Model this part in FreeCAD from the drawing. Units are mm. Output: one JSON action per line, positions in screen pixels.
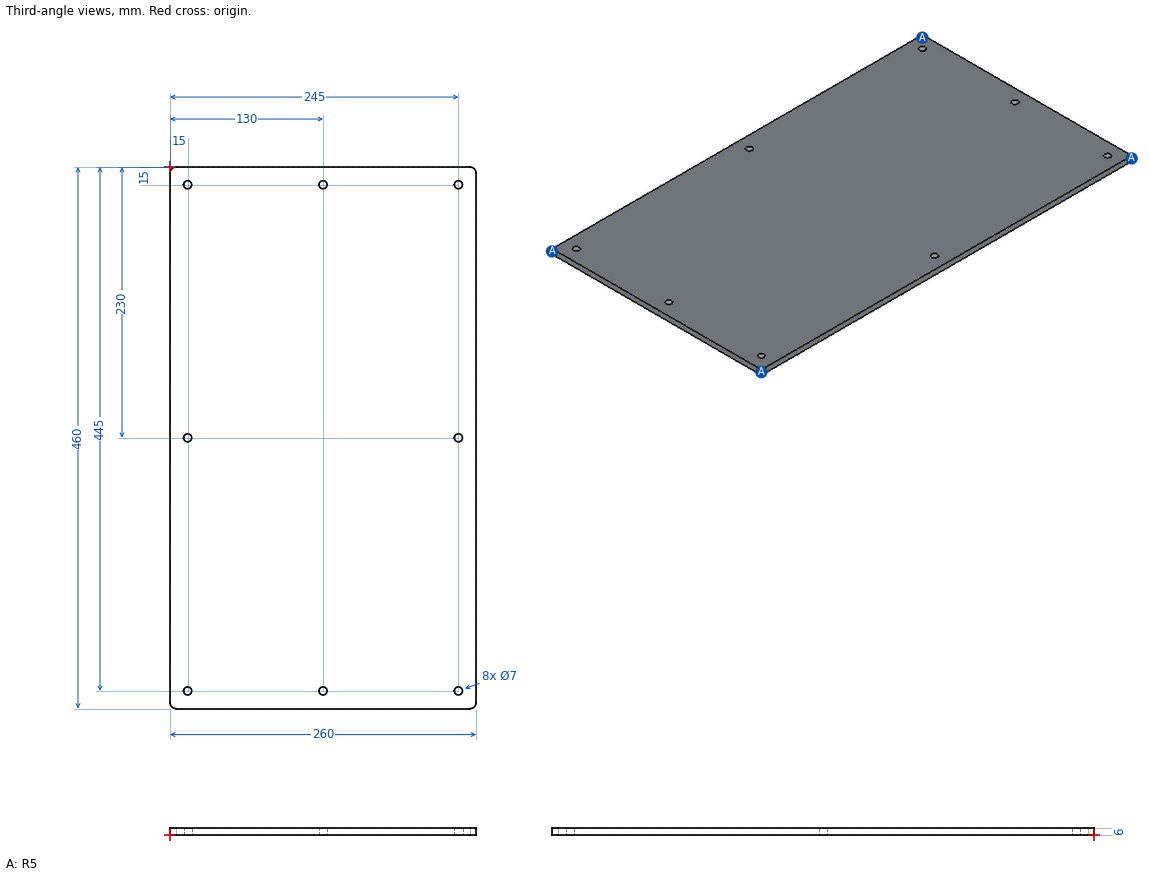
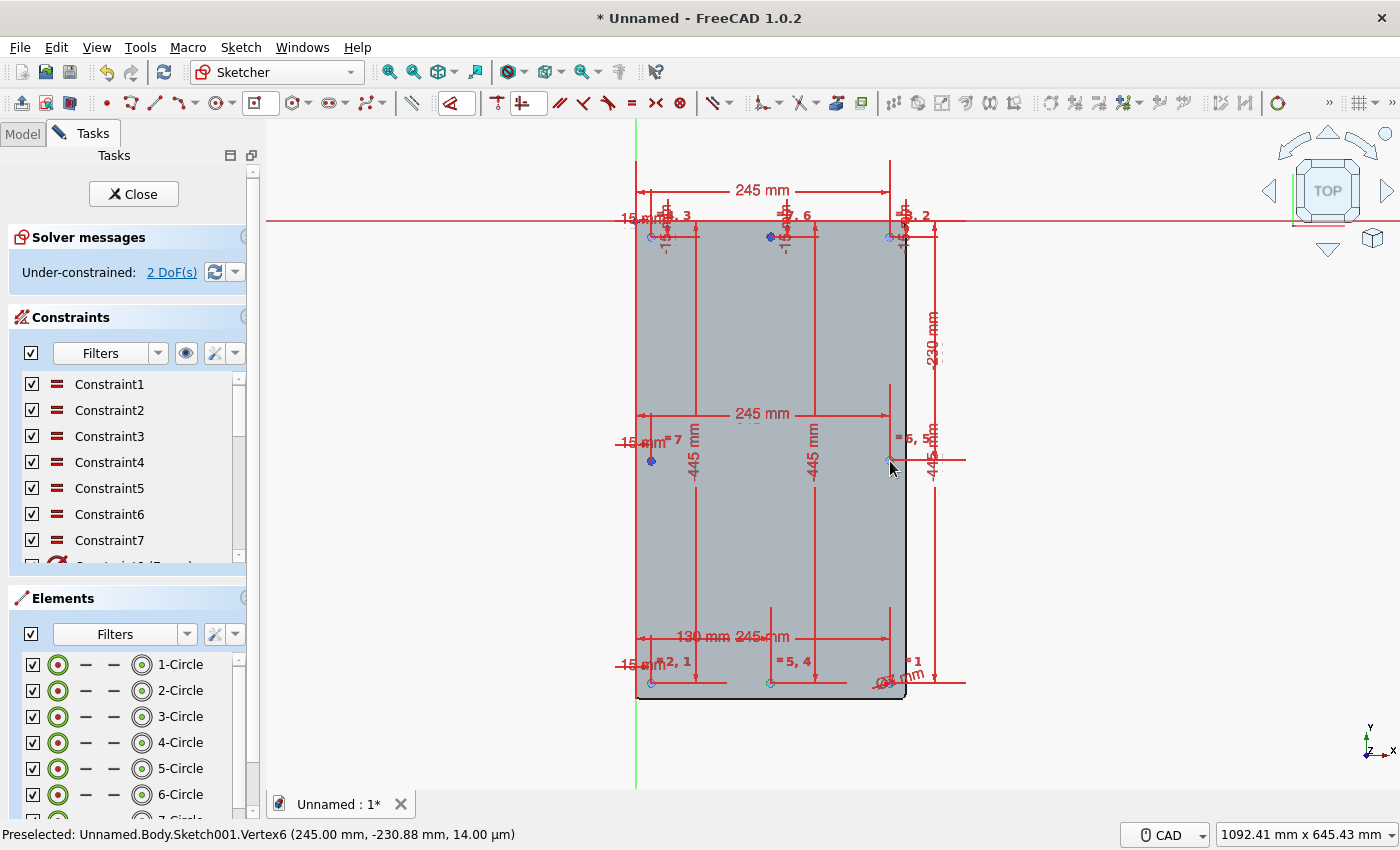
{"action": "left_click", "coordinate": [771, 237]}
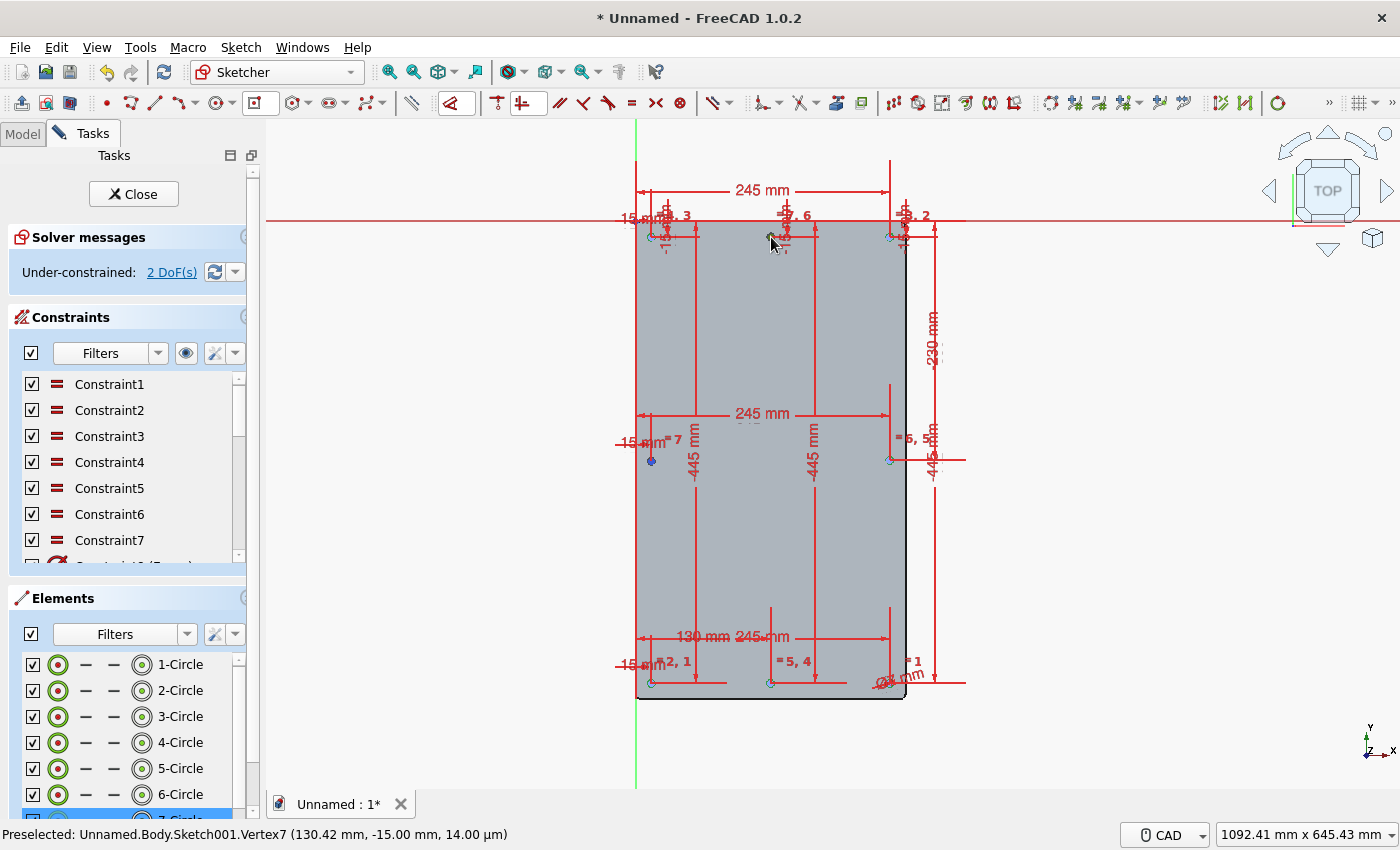
{"action": "key", "text": "l"}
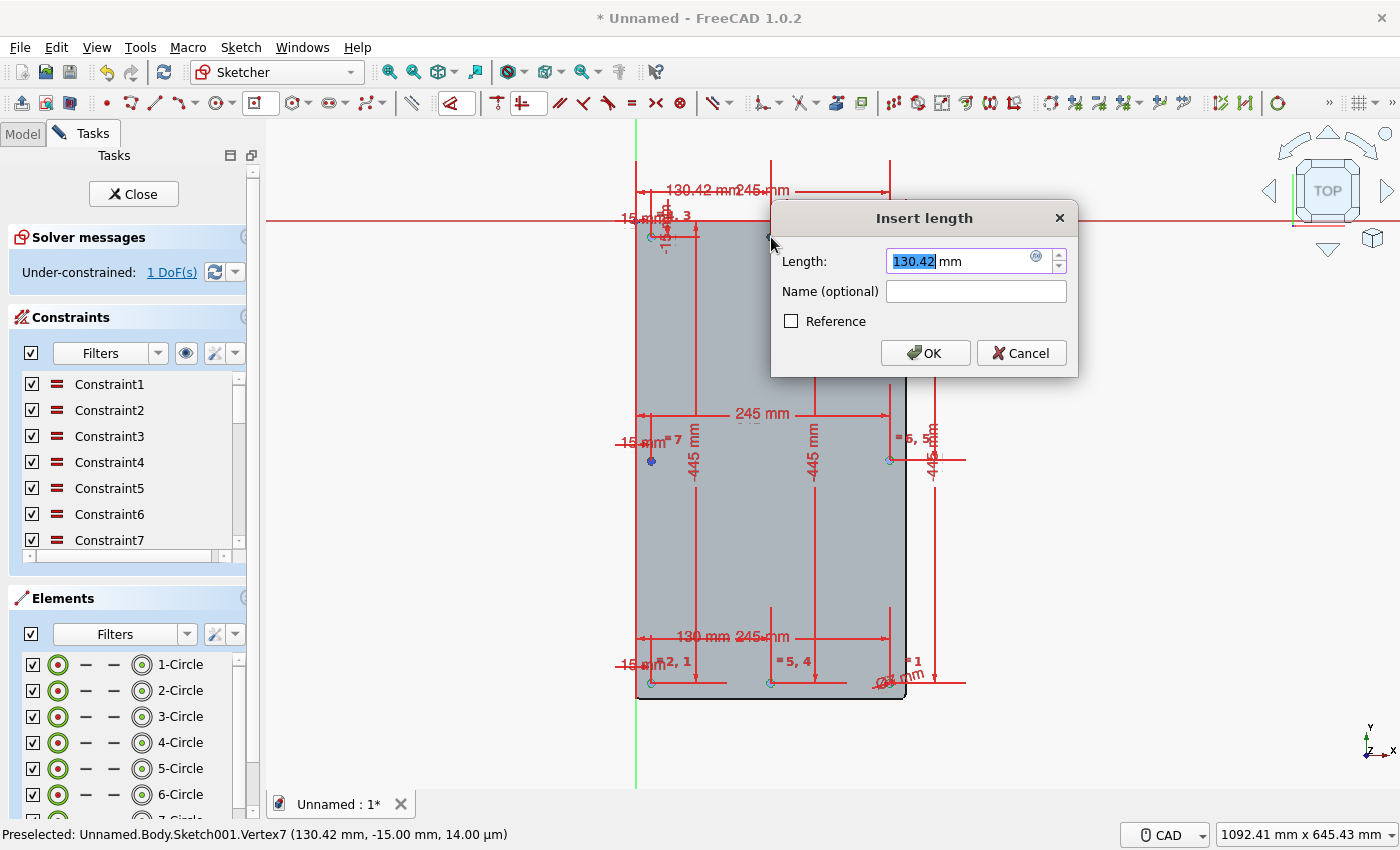
{"action": "type", "text": "130"}
{"action": "key", "text": "Return"}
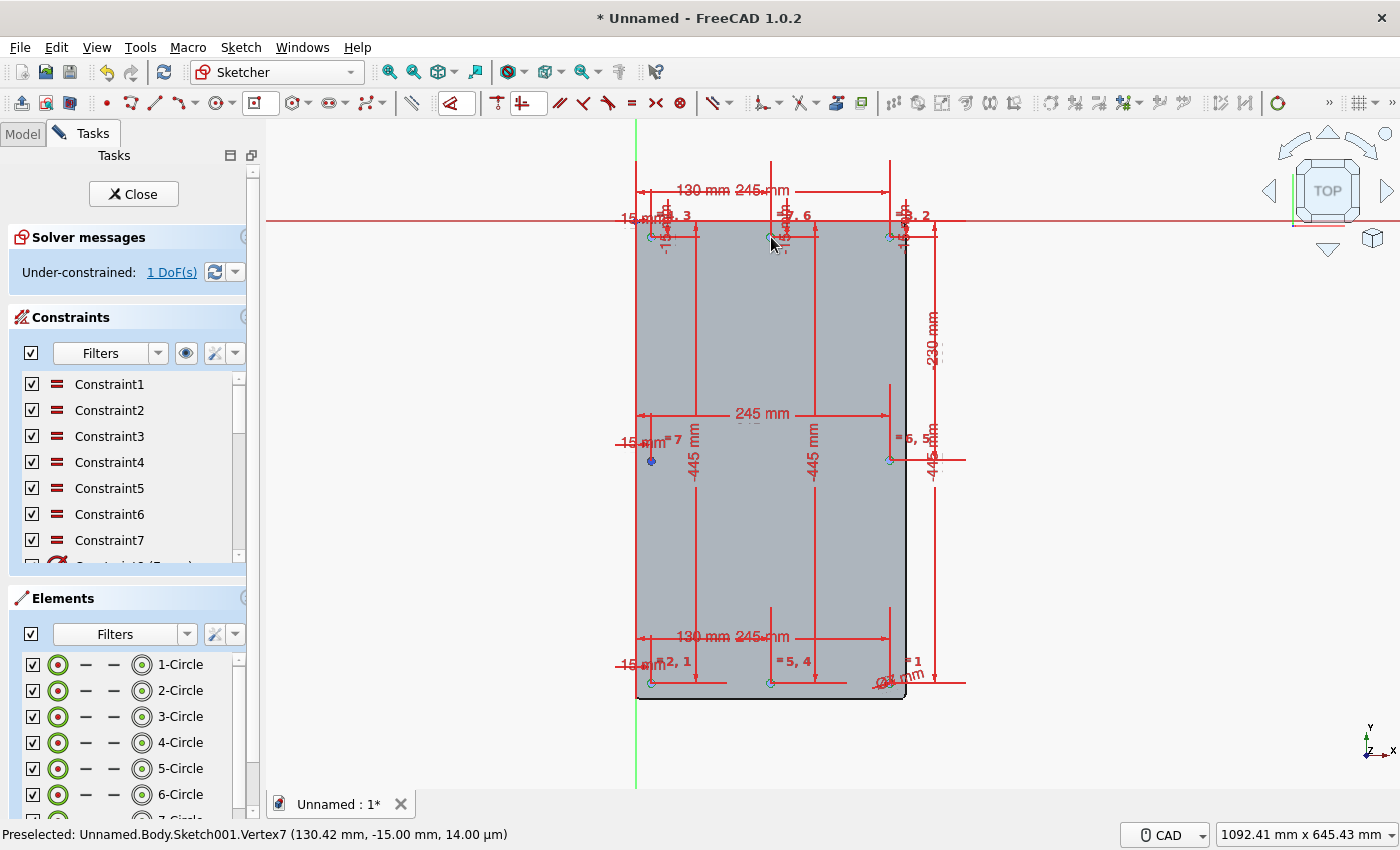
{"action": "left_click", "coordinate": [651, 461]}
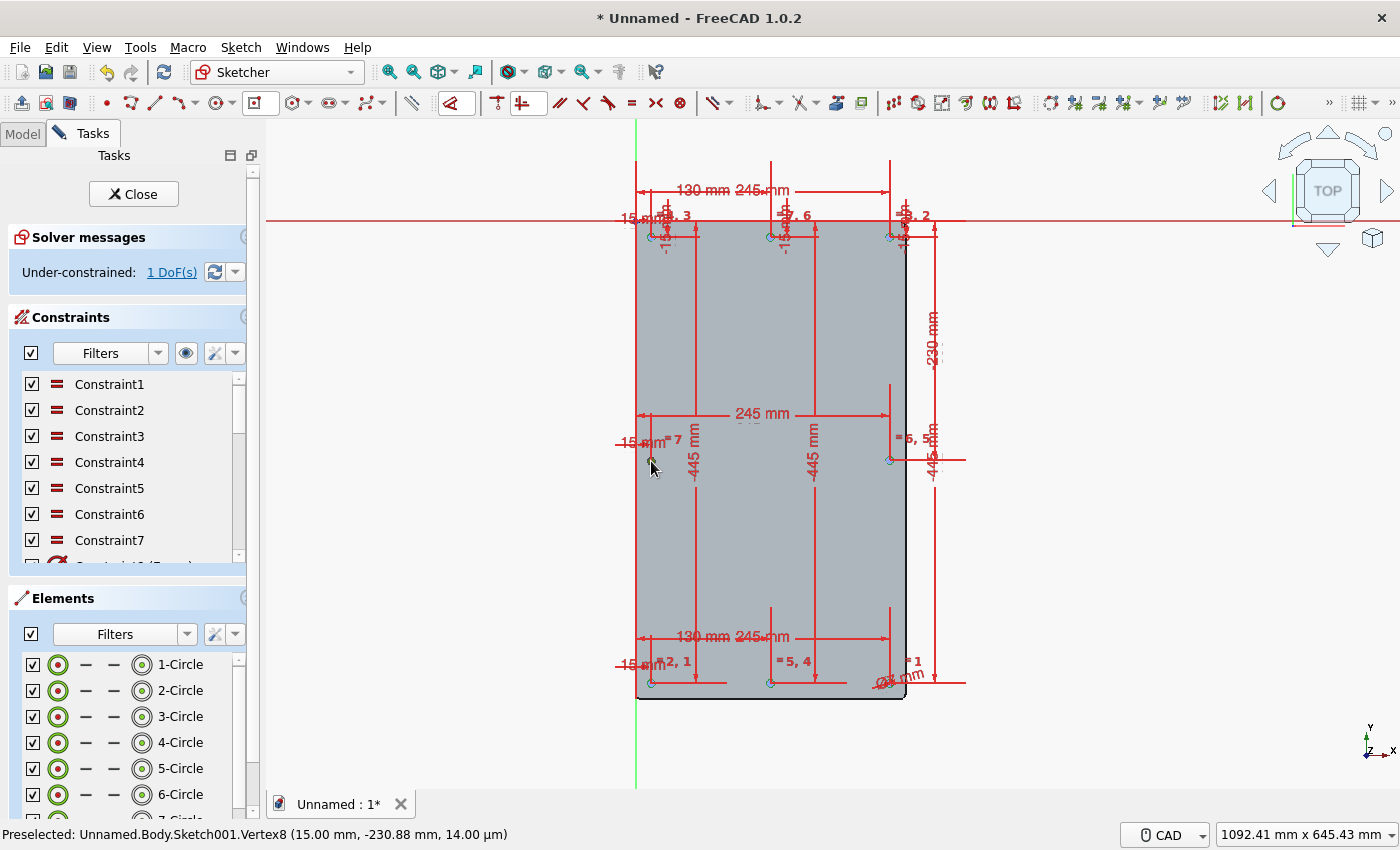
{"action": "left_click", "coordinate": [470, 104]}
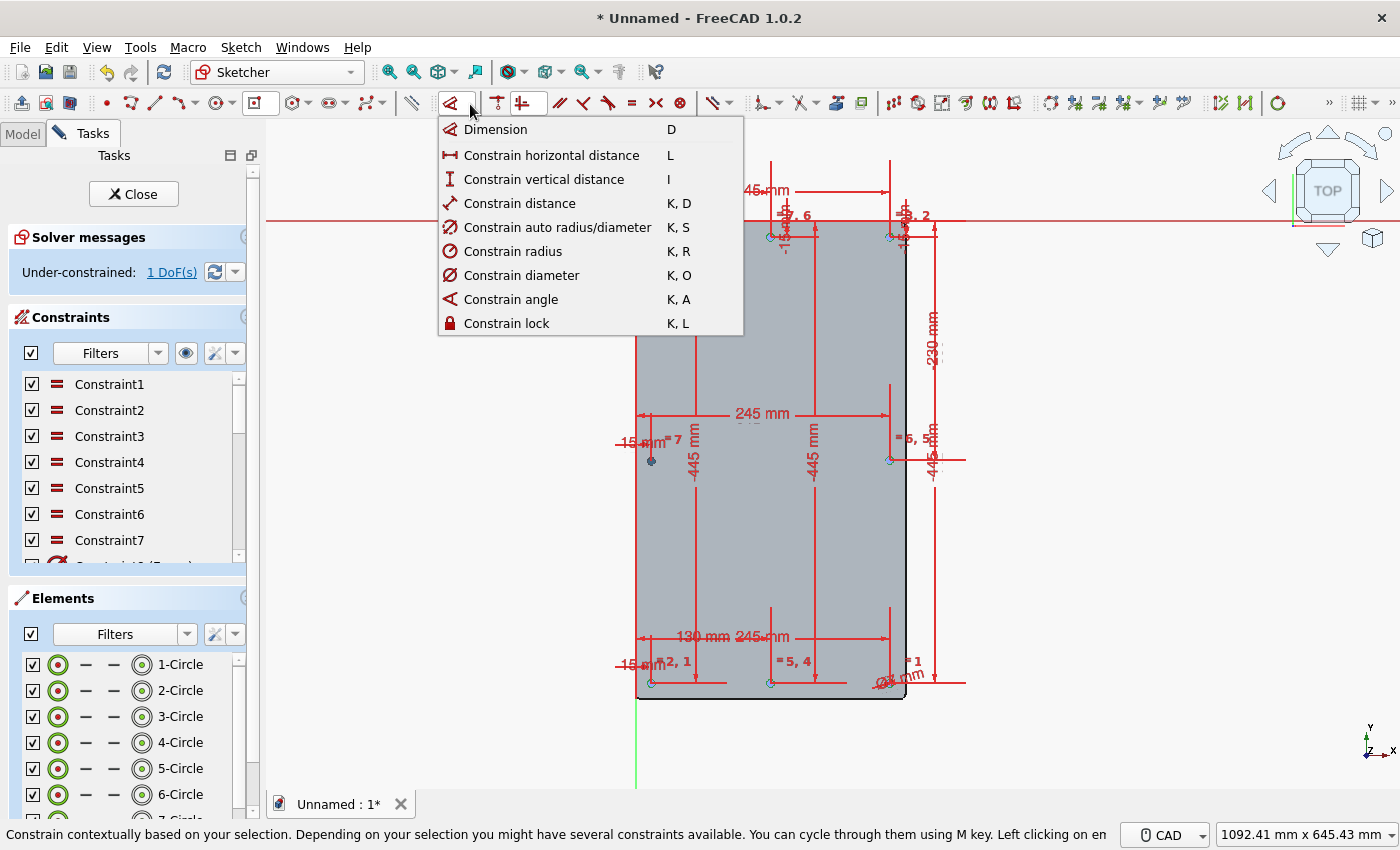
{"action": "left_click", "coordinate": [591, 179]}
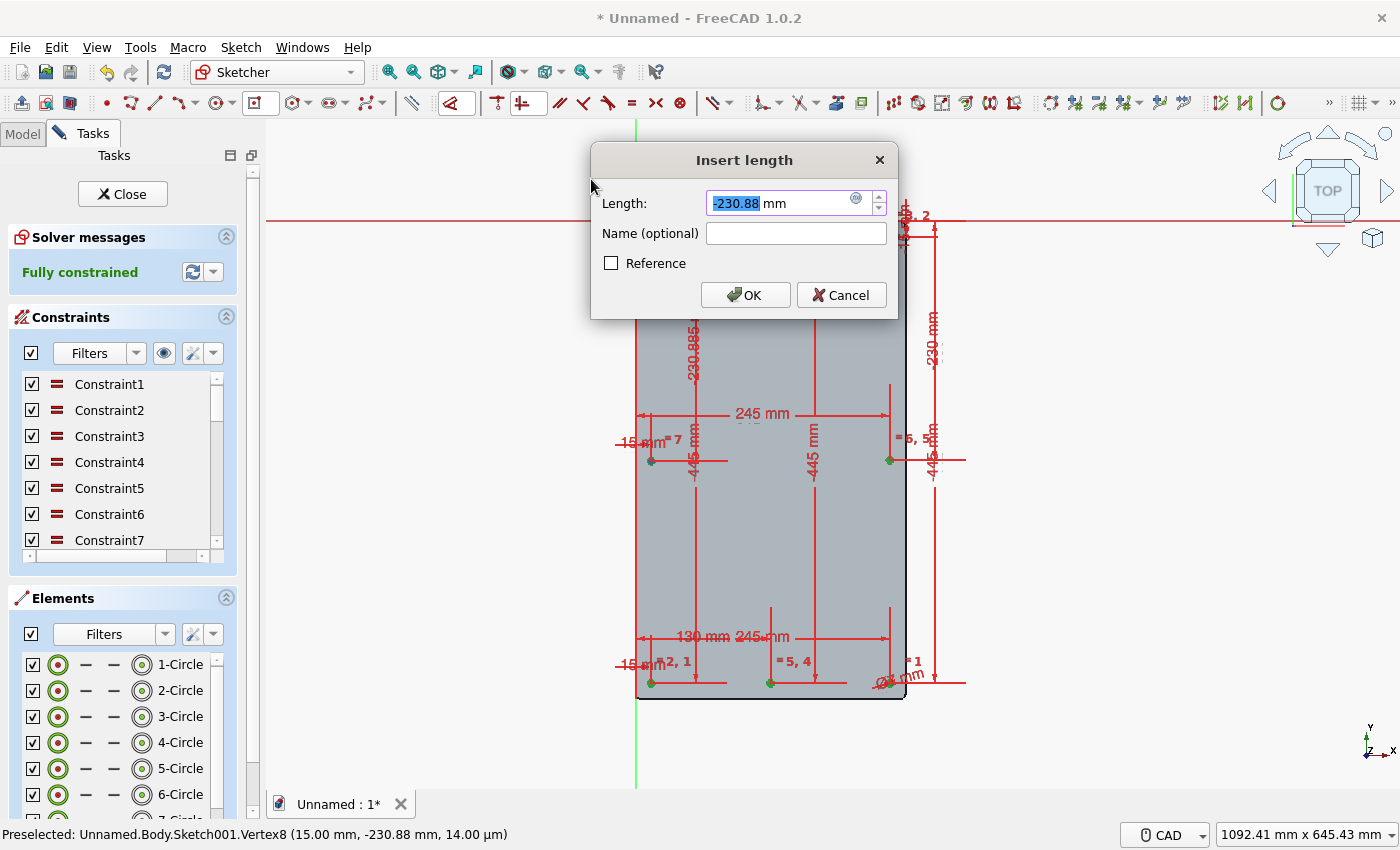
{"action": "type", "text": "-230"}
{"action": "key", "text": "Return"}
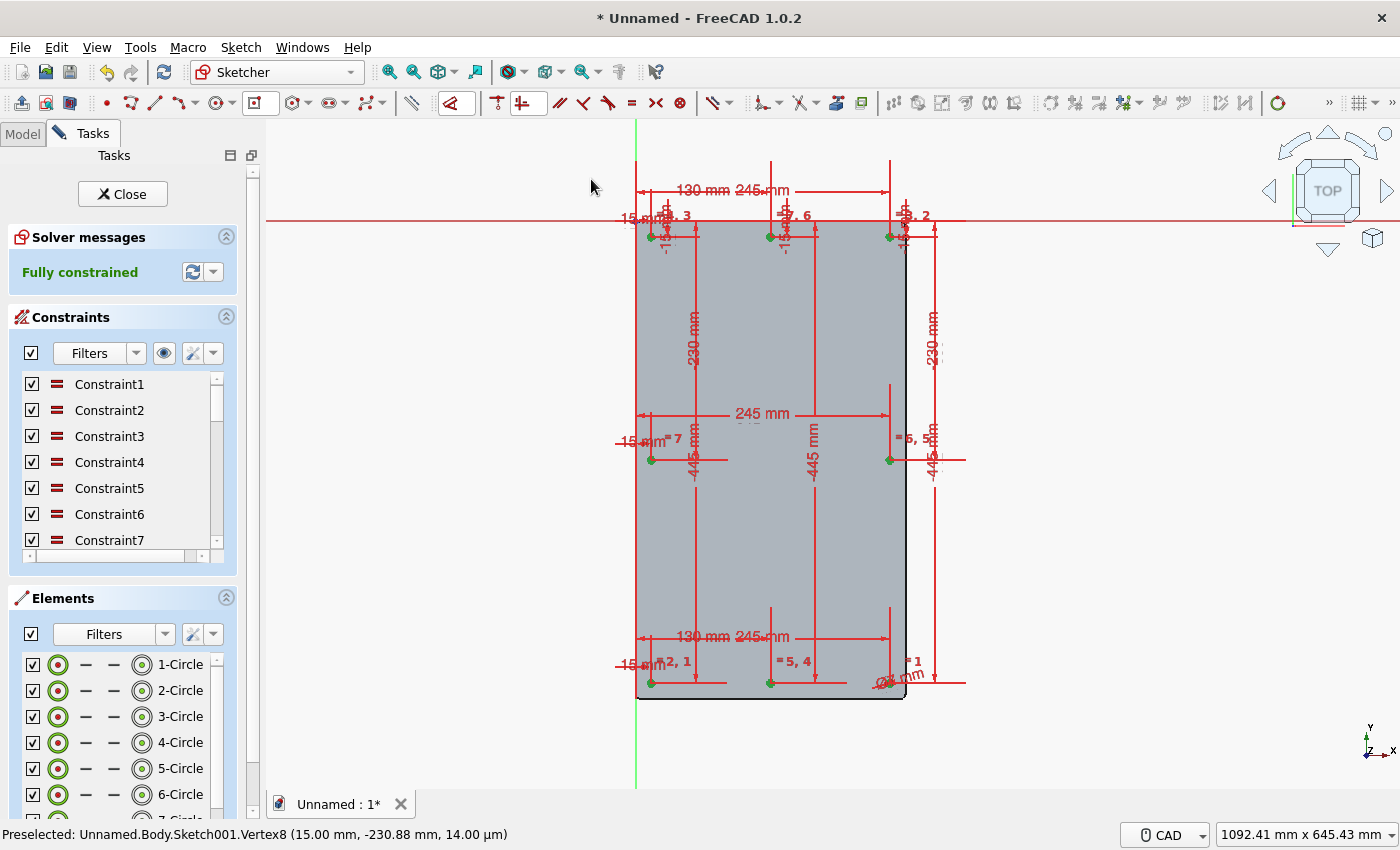
{"action": "left_click", "coordinate": [123, 194]}